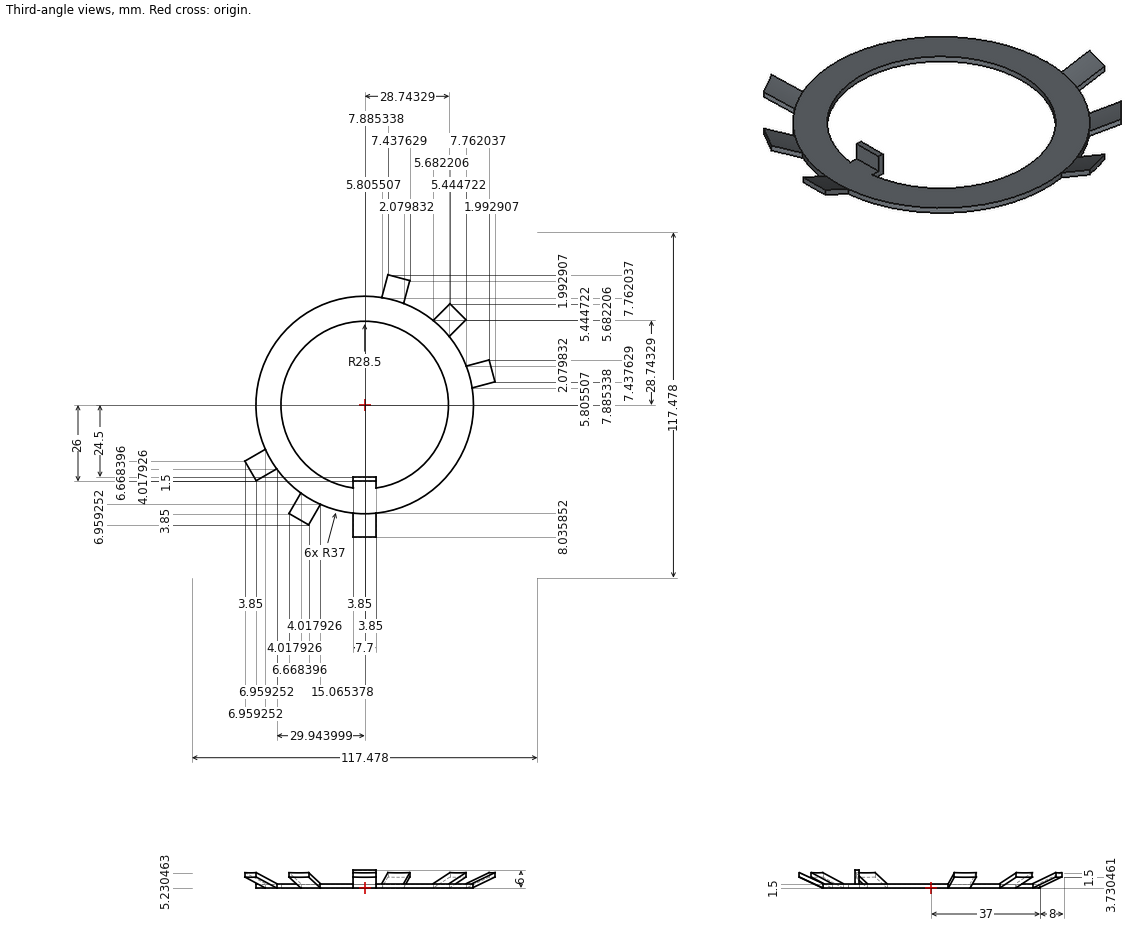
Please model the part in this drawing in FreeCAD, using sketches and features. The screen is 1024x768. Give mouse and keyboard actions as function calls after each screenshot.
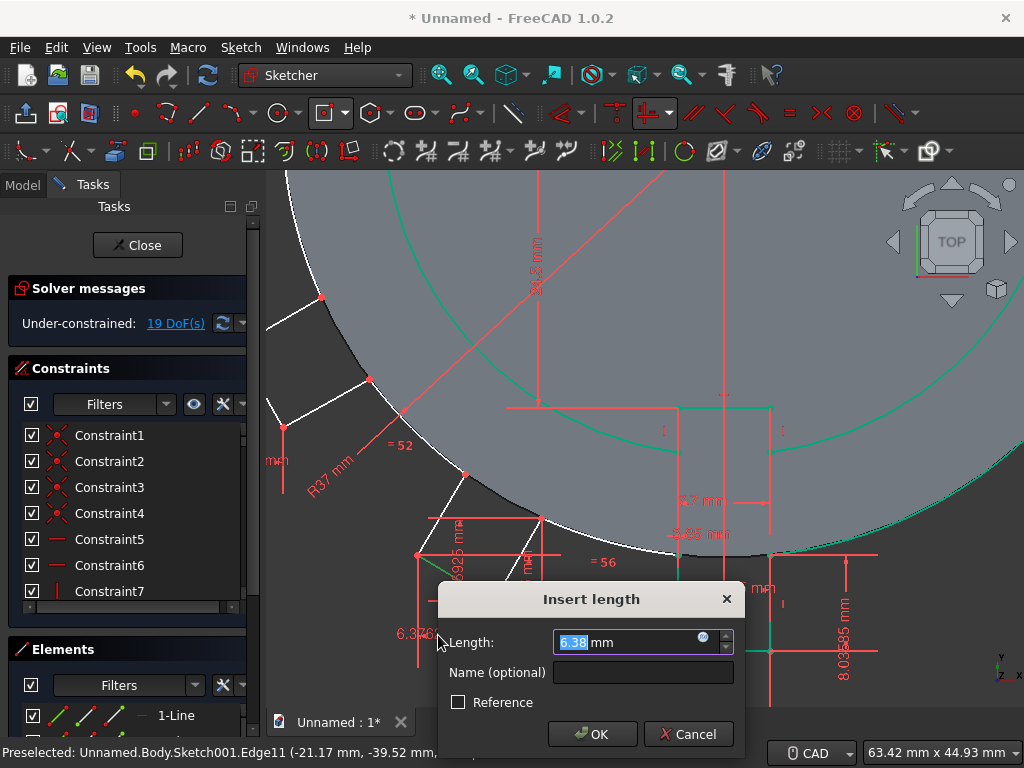
text(6.668396)
key(Return)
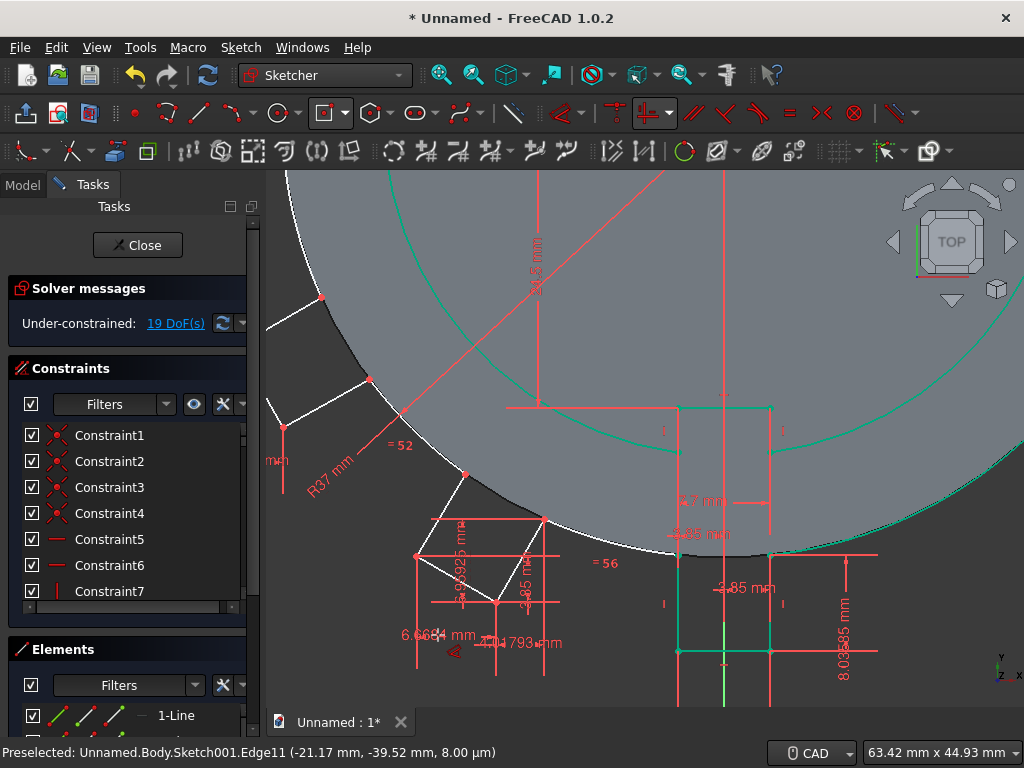
click(431, 532)
click(441, 590)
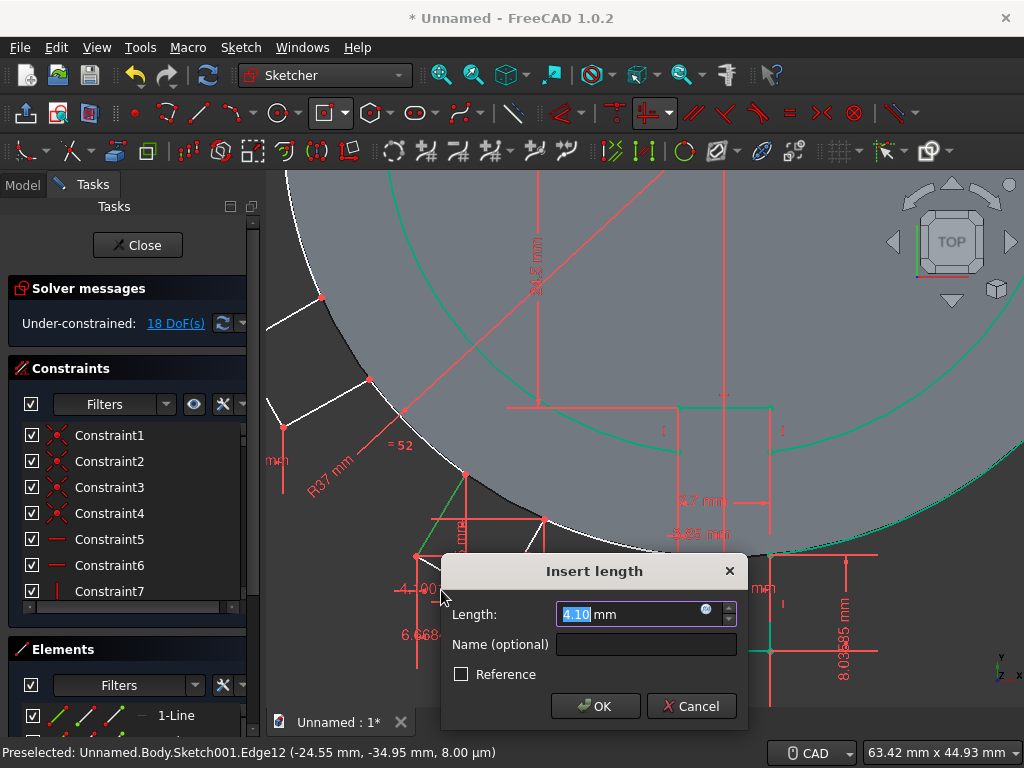
text(4.017926)
key(Return)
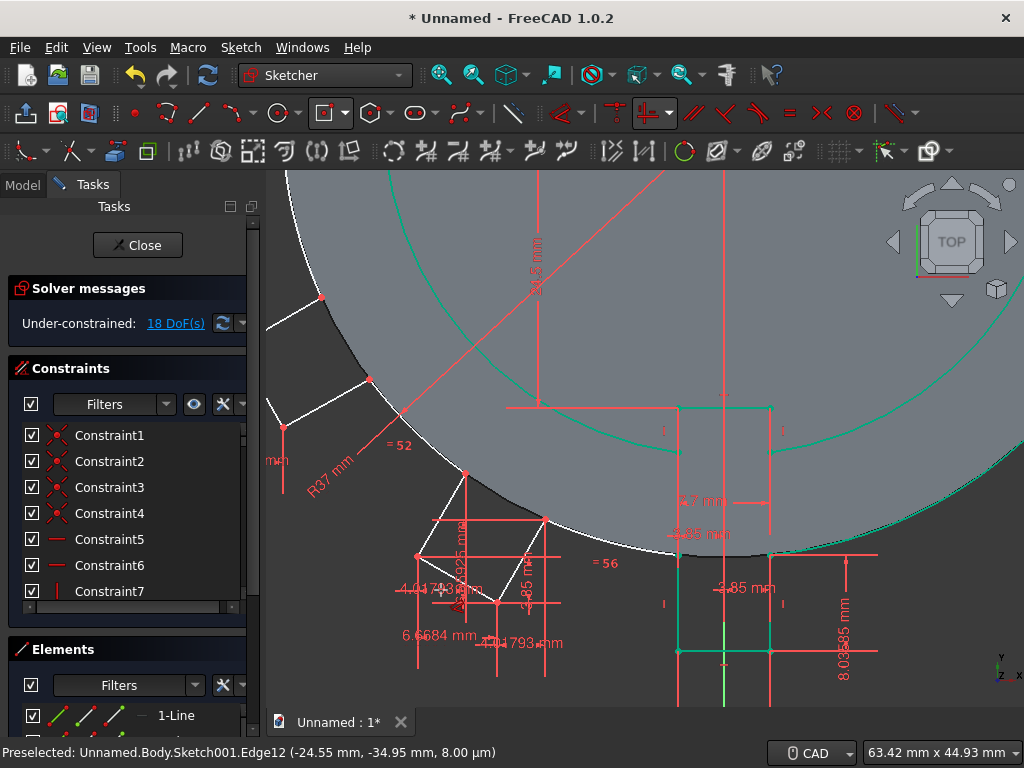
click(344, 394)
click(332, 345)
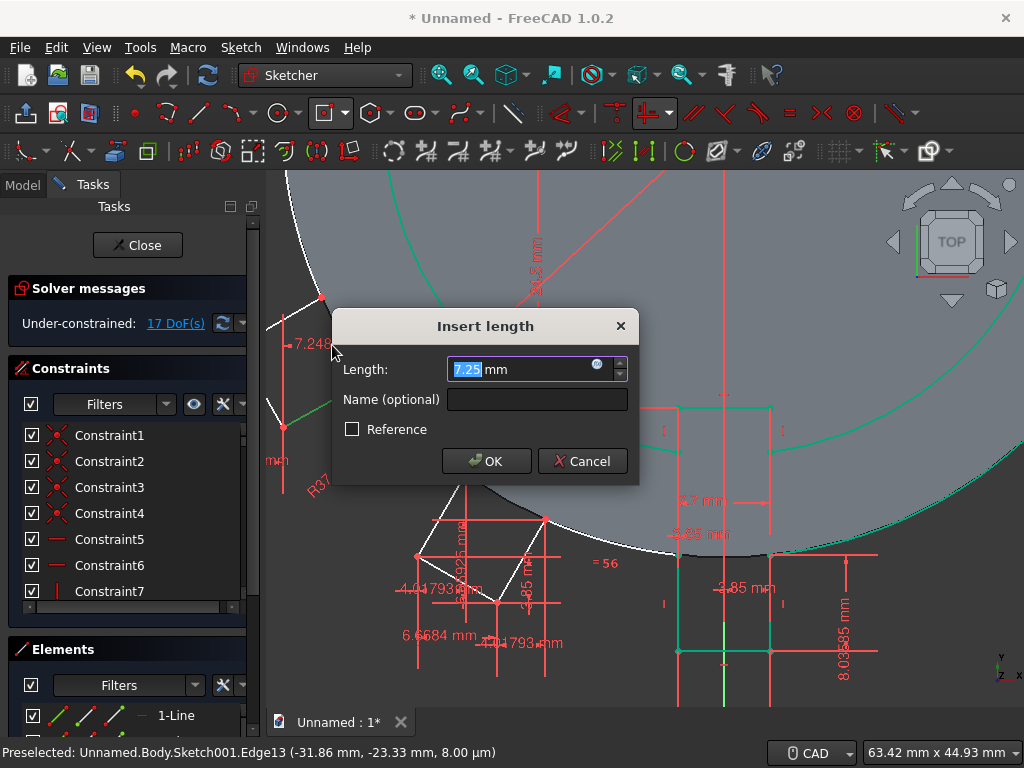
text(6.959252)
key(Return)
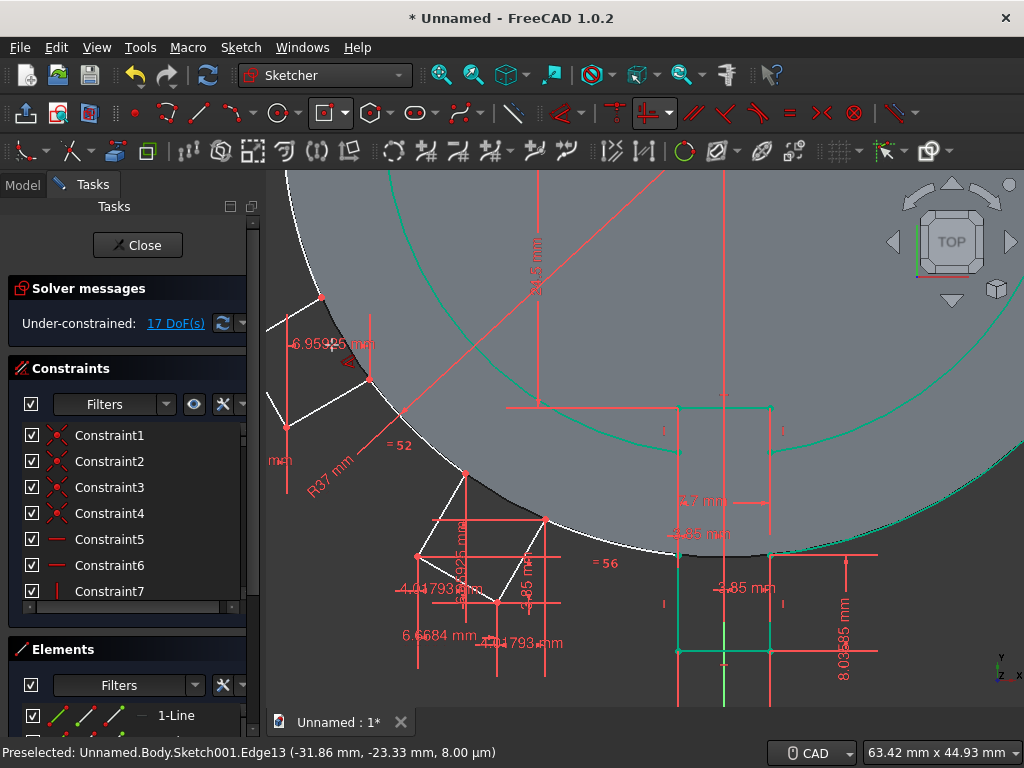
click(345, 394)
click(404, 393)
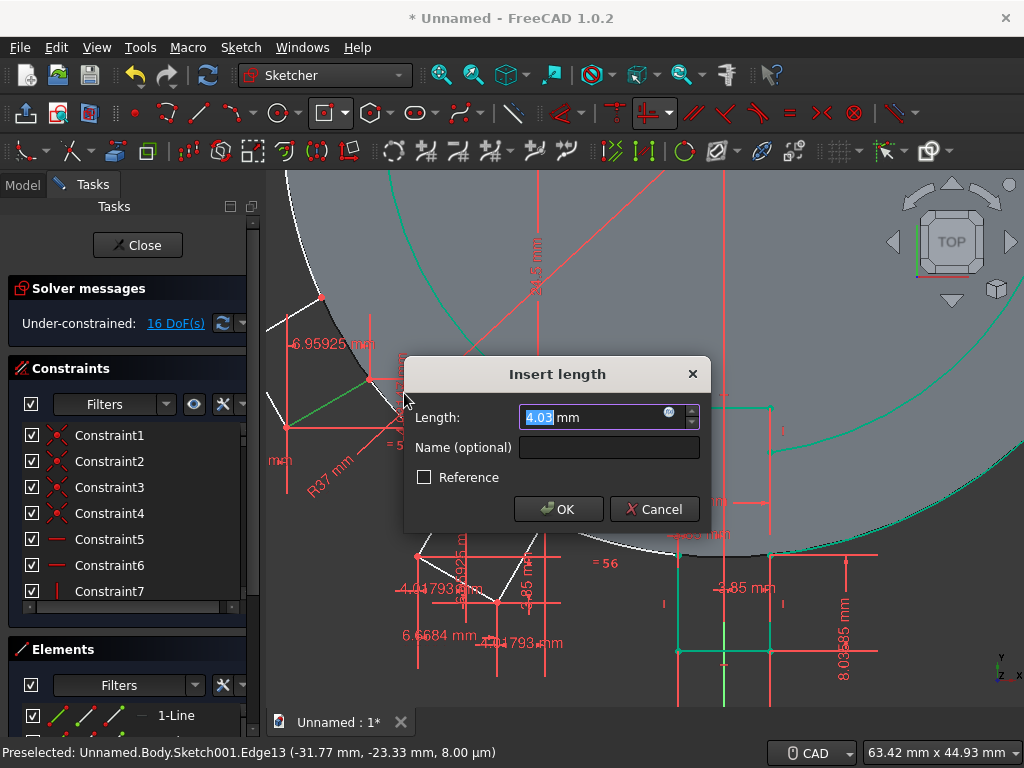
text(4.017926)
key(Return)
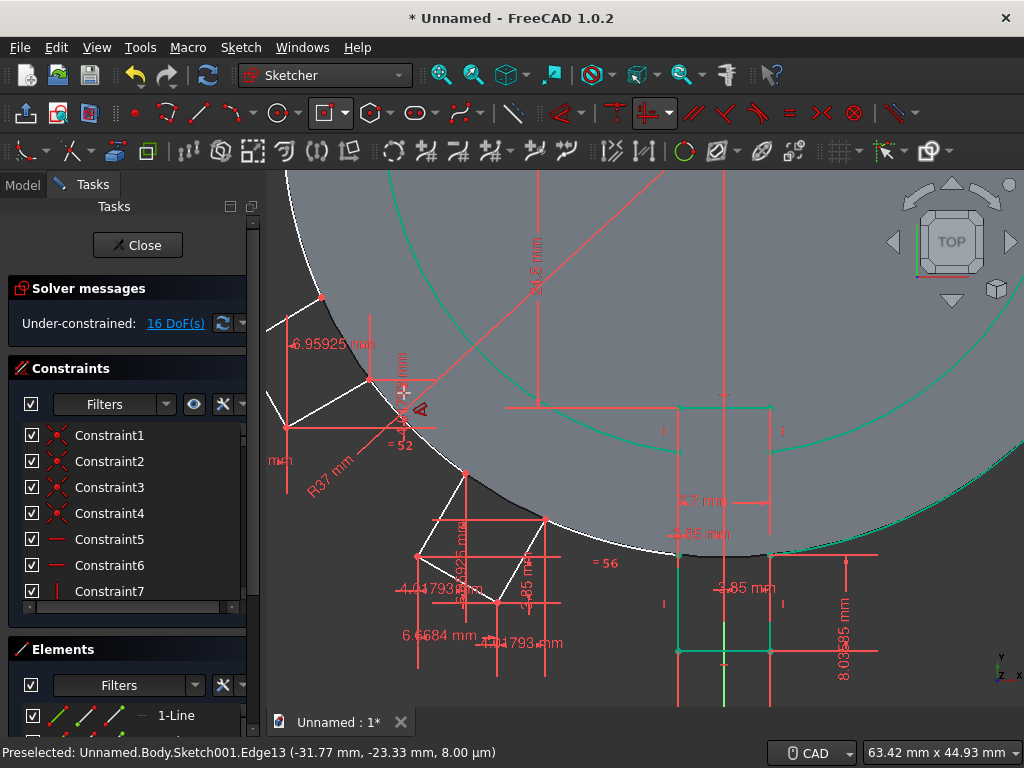
scroll(528, 544, down, 7)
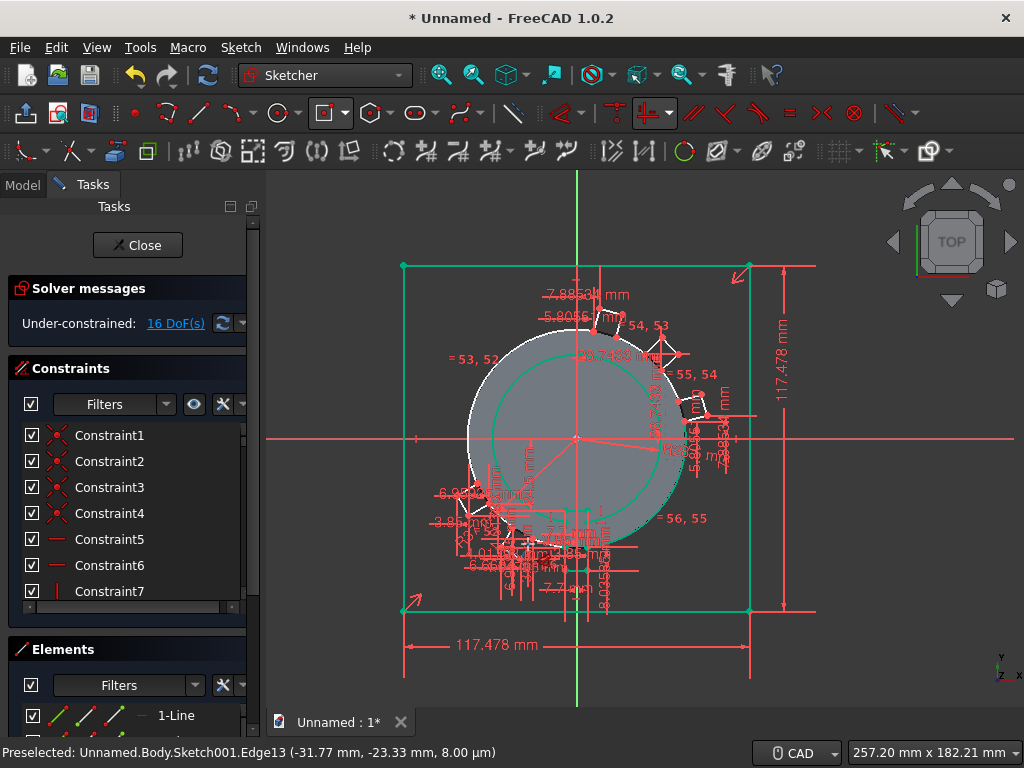
scroll(465, 510, up, 4)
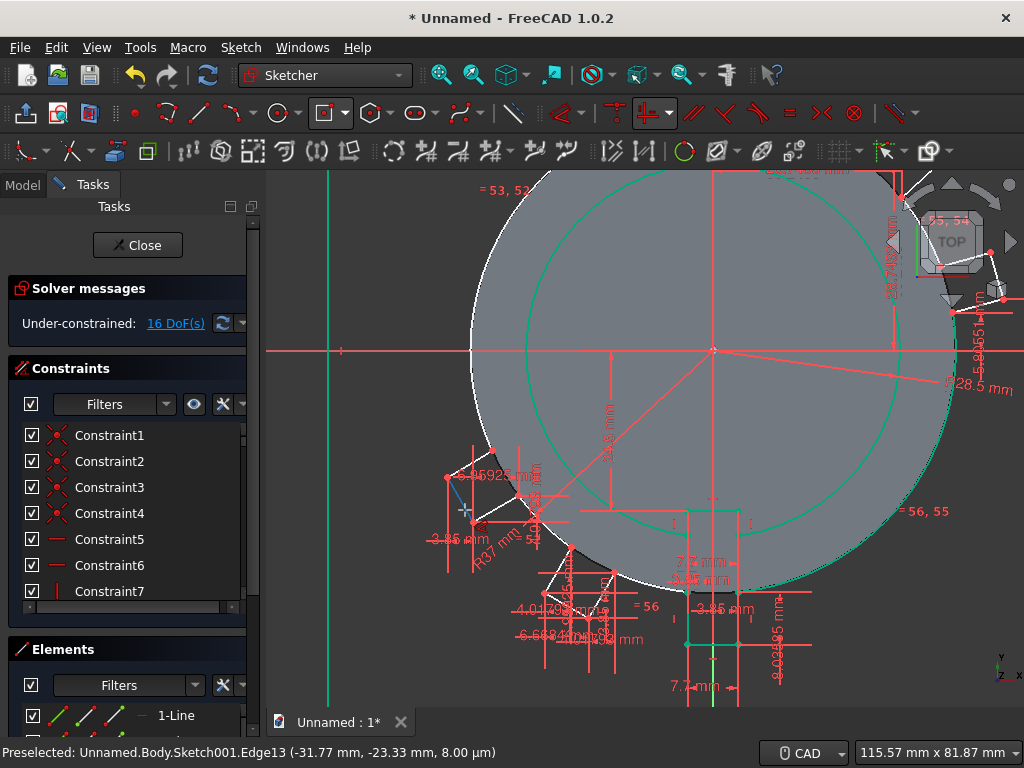
click(465, 509)
click(414, 500)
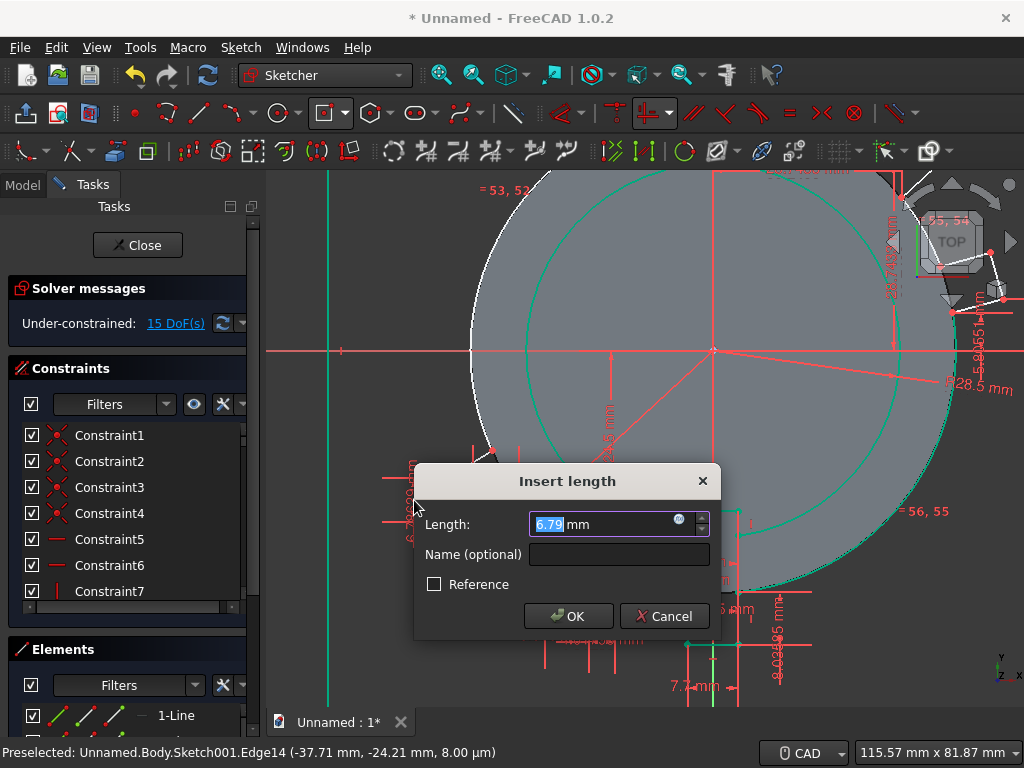
text(6.668396)
key(Return)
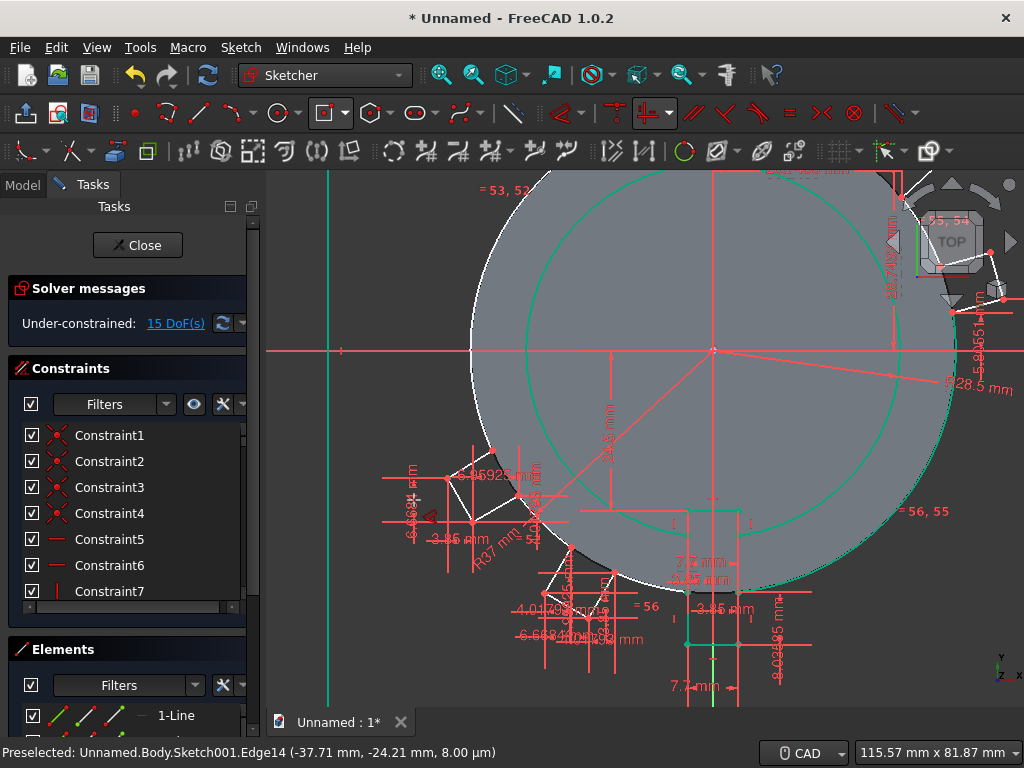
click(461, 470)
click(460, 417)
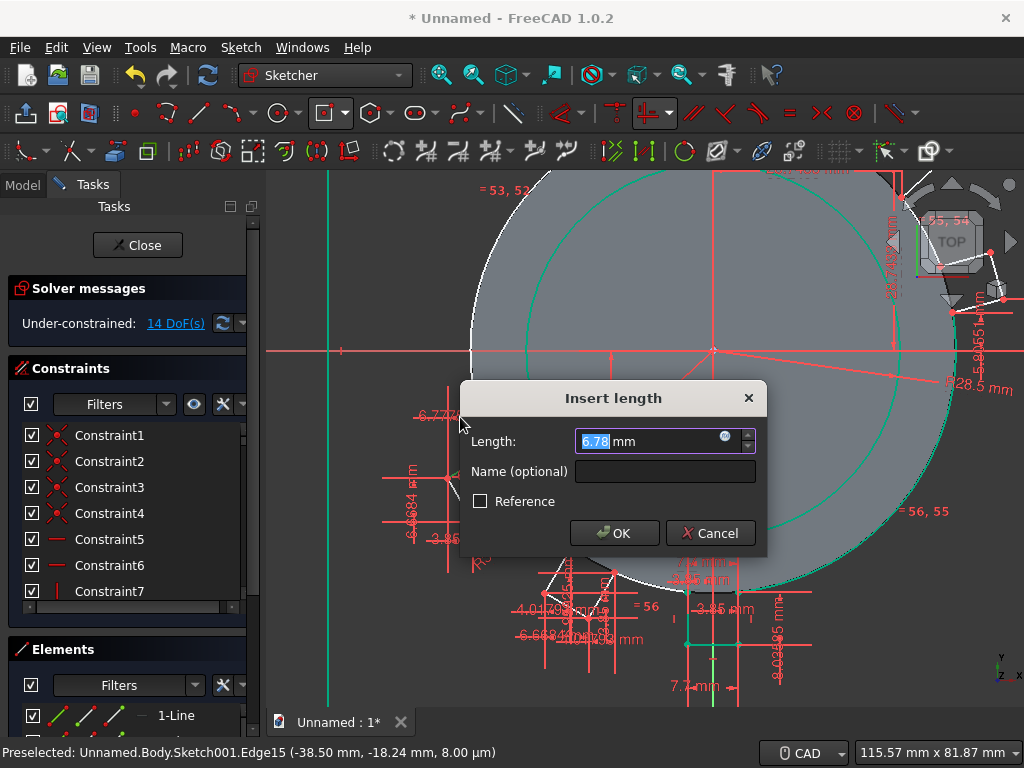
text(6.959252)
key(Return)